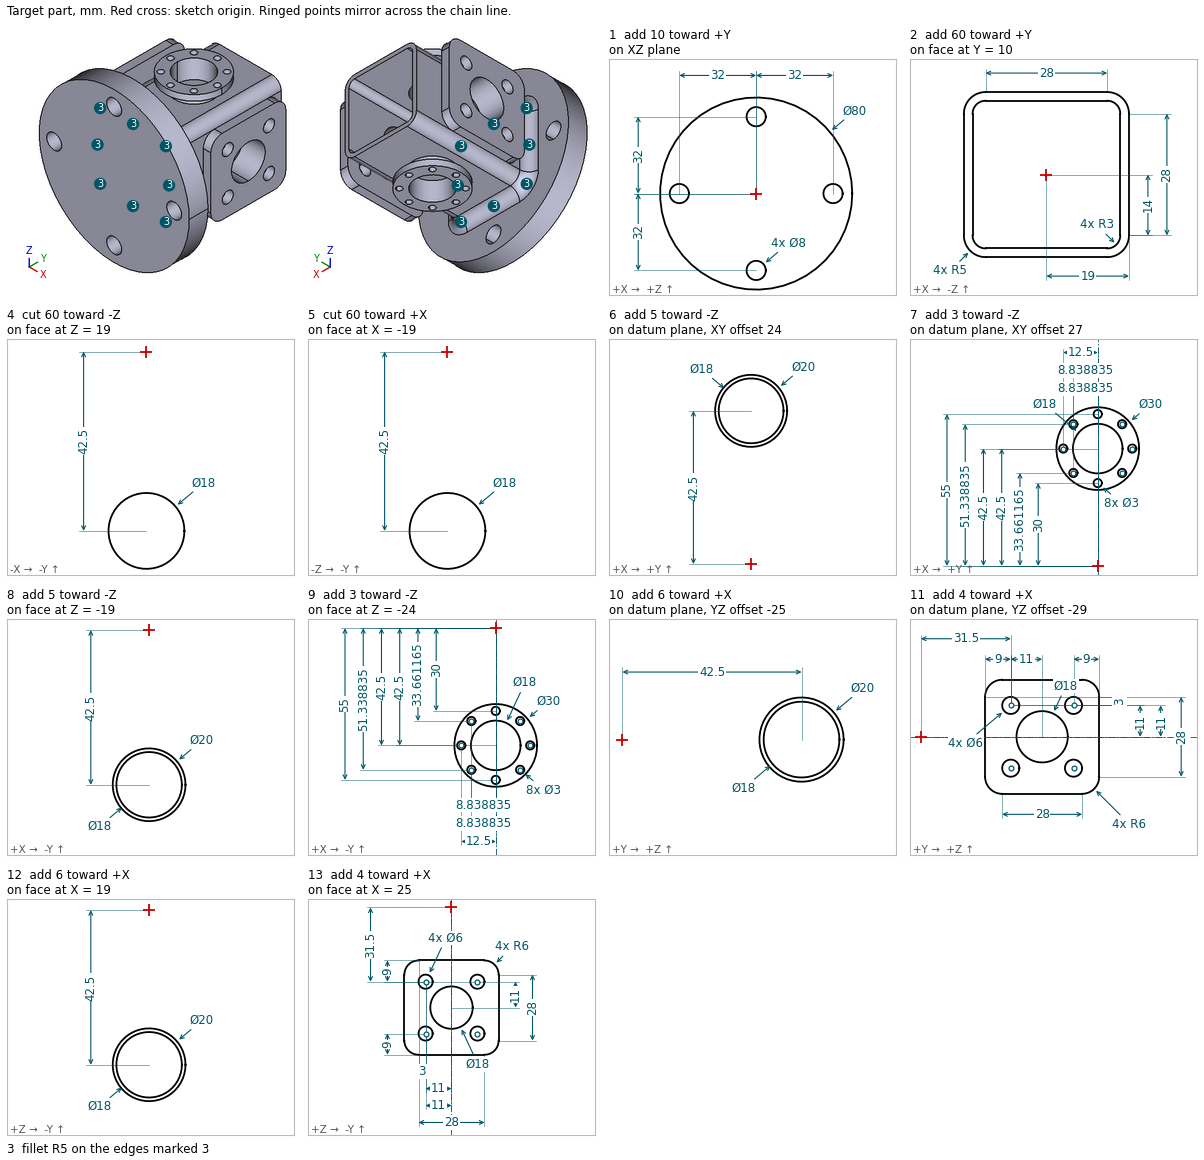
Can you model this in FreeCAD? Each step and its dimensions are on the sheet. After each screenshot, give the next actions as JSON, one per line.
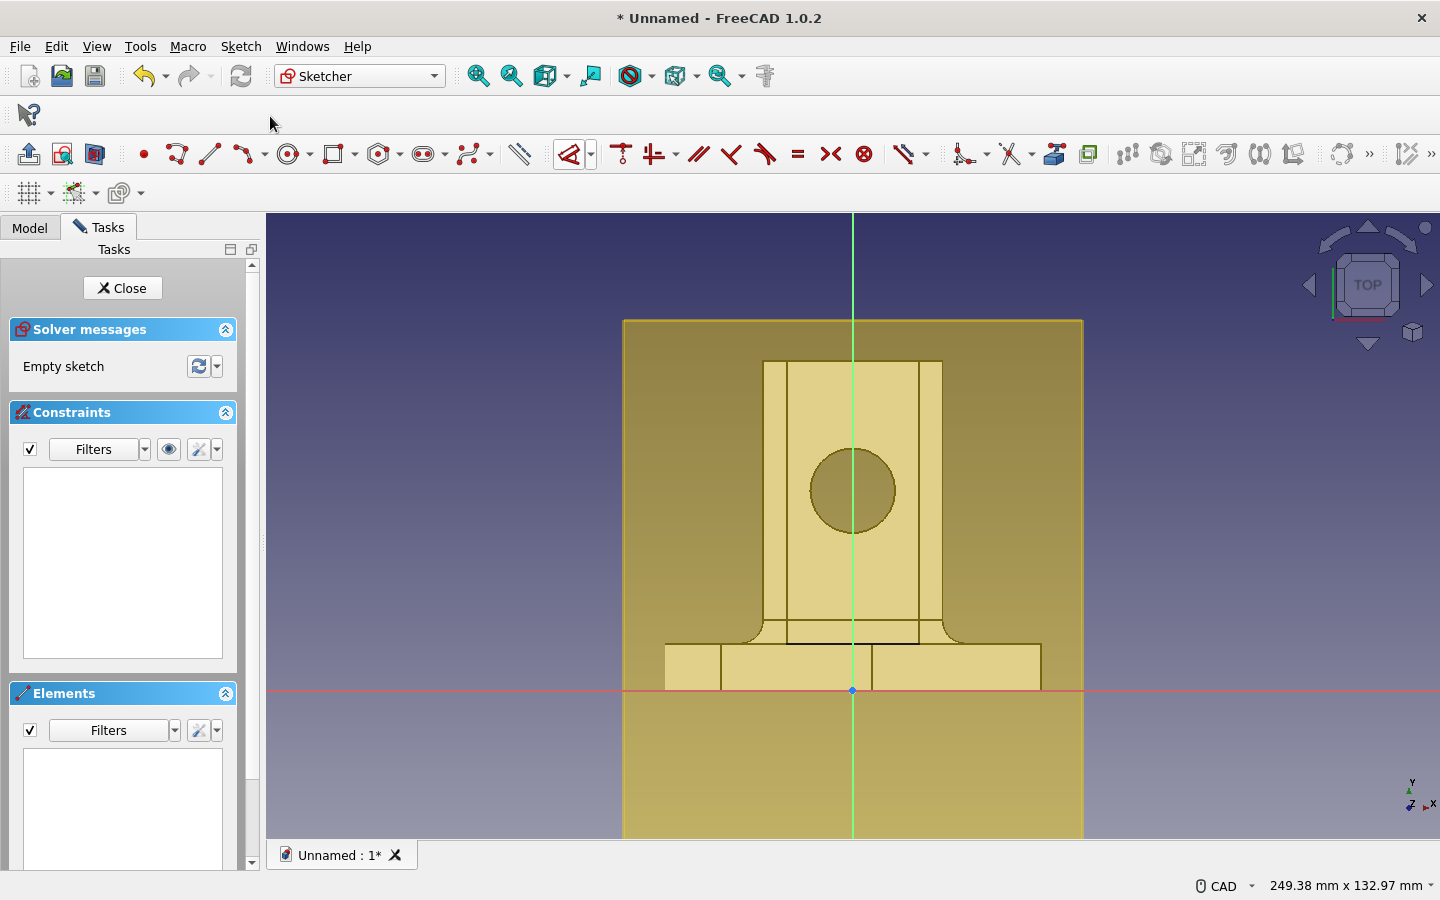
{"action": "scroll", "coordinate": [875, 479], "scroll_direction": "up", "scroll_amount": 7}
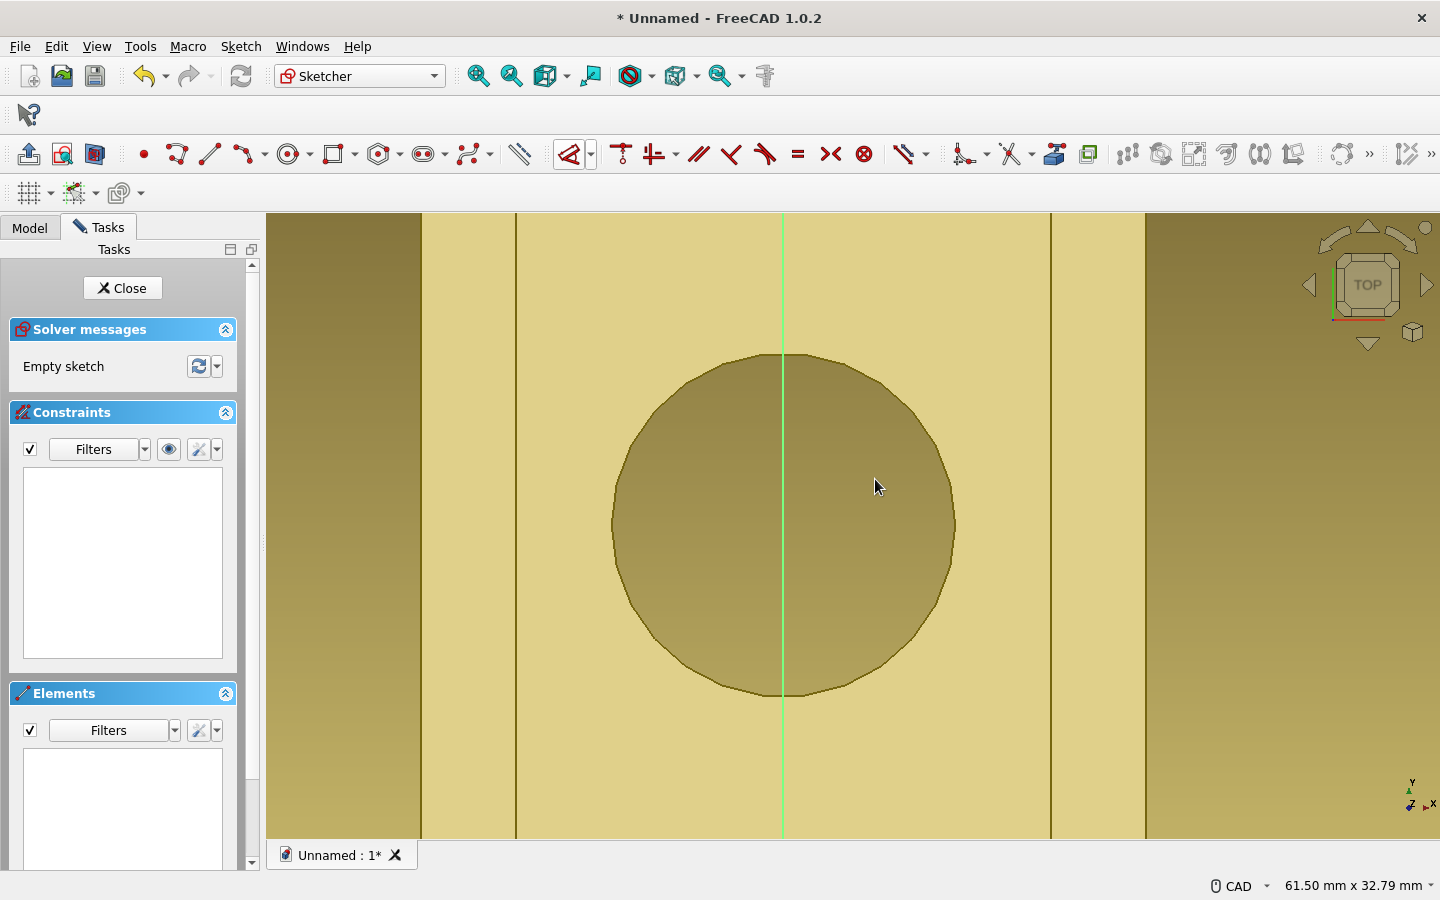
{"action": "key", "text": "g c"}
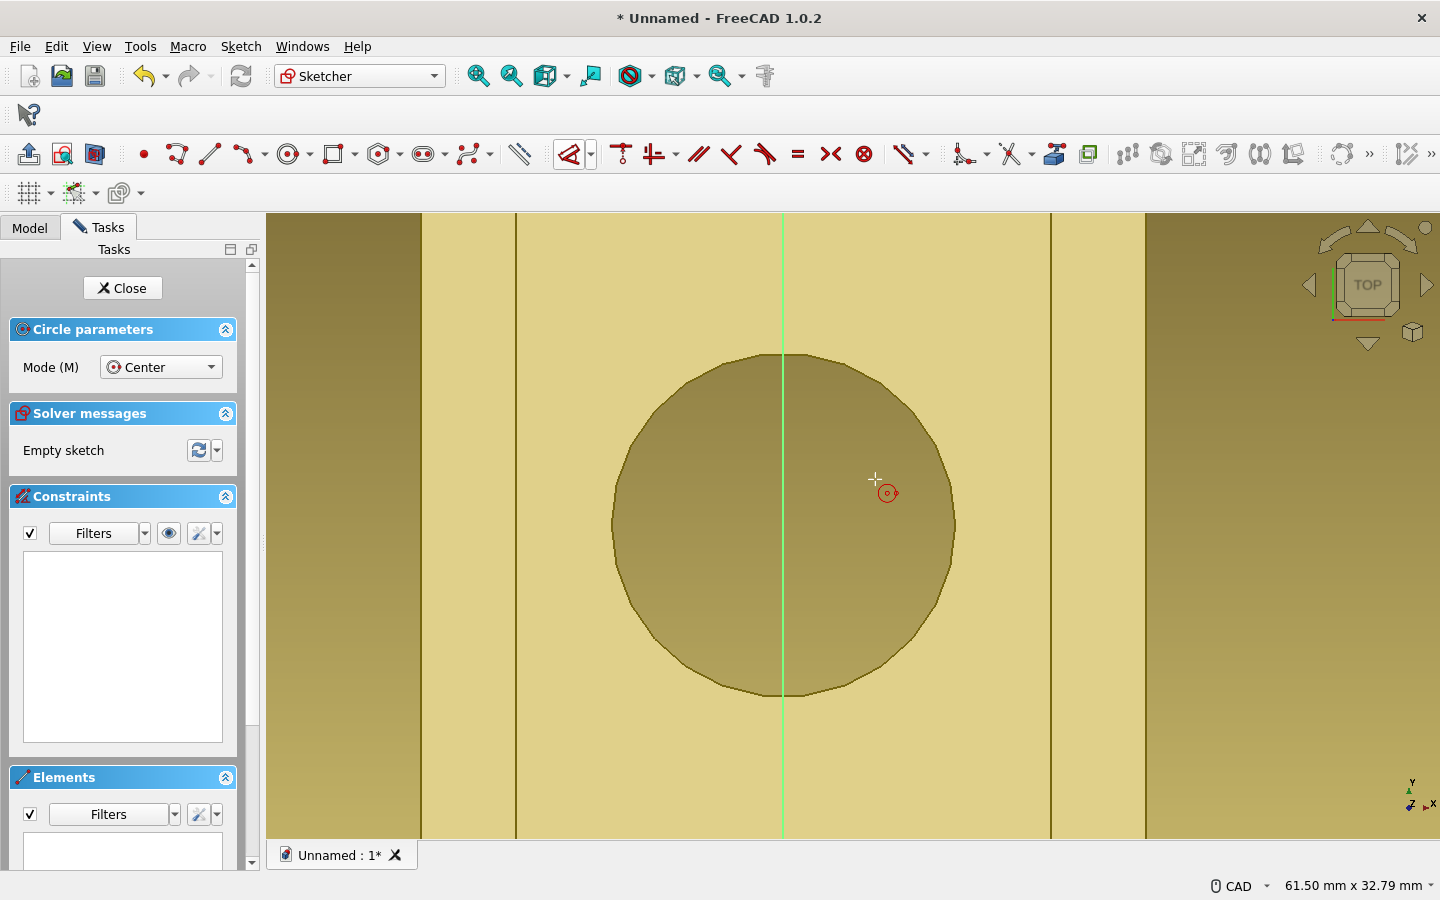
{"action": "left_click", "coordinate": [783, 525]}
{"action": "mouse_move", "coordinate": [918, 390]}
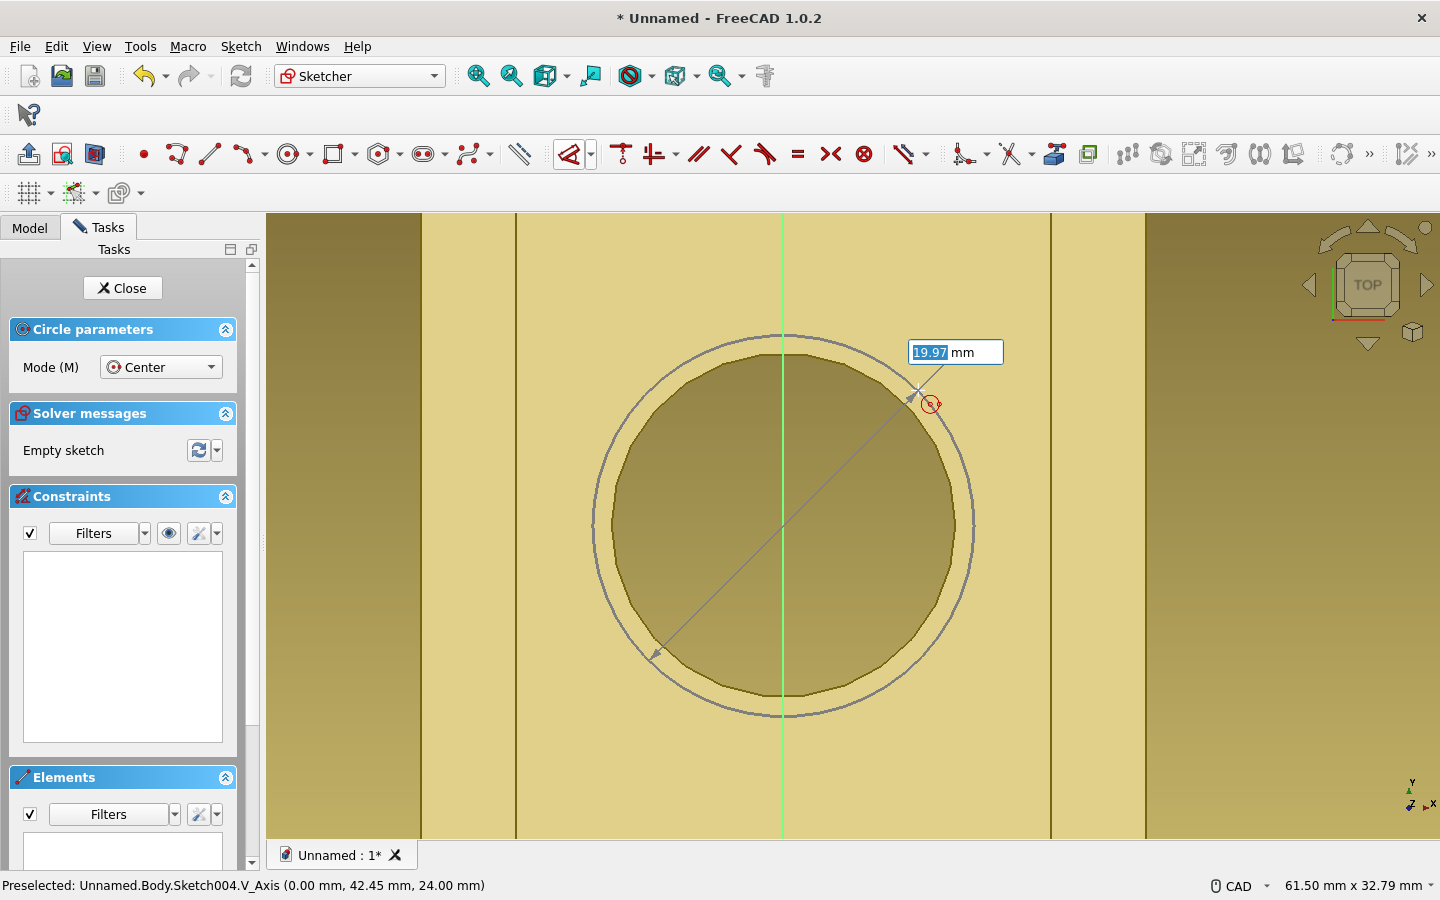
{"action": "type", "text": "20"}
{"action": "key", "text": "Return"}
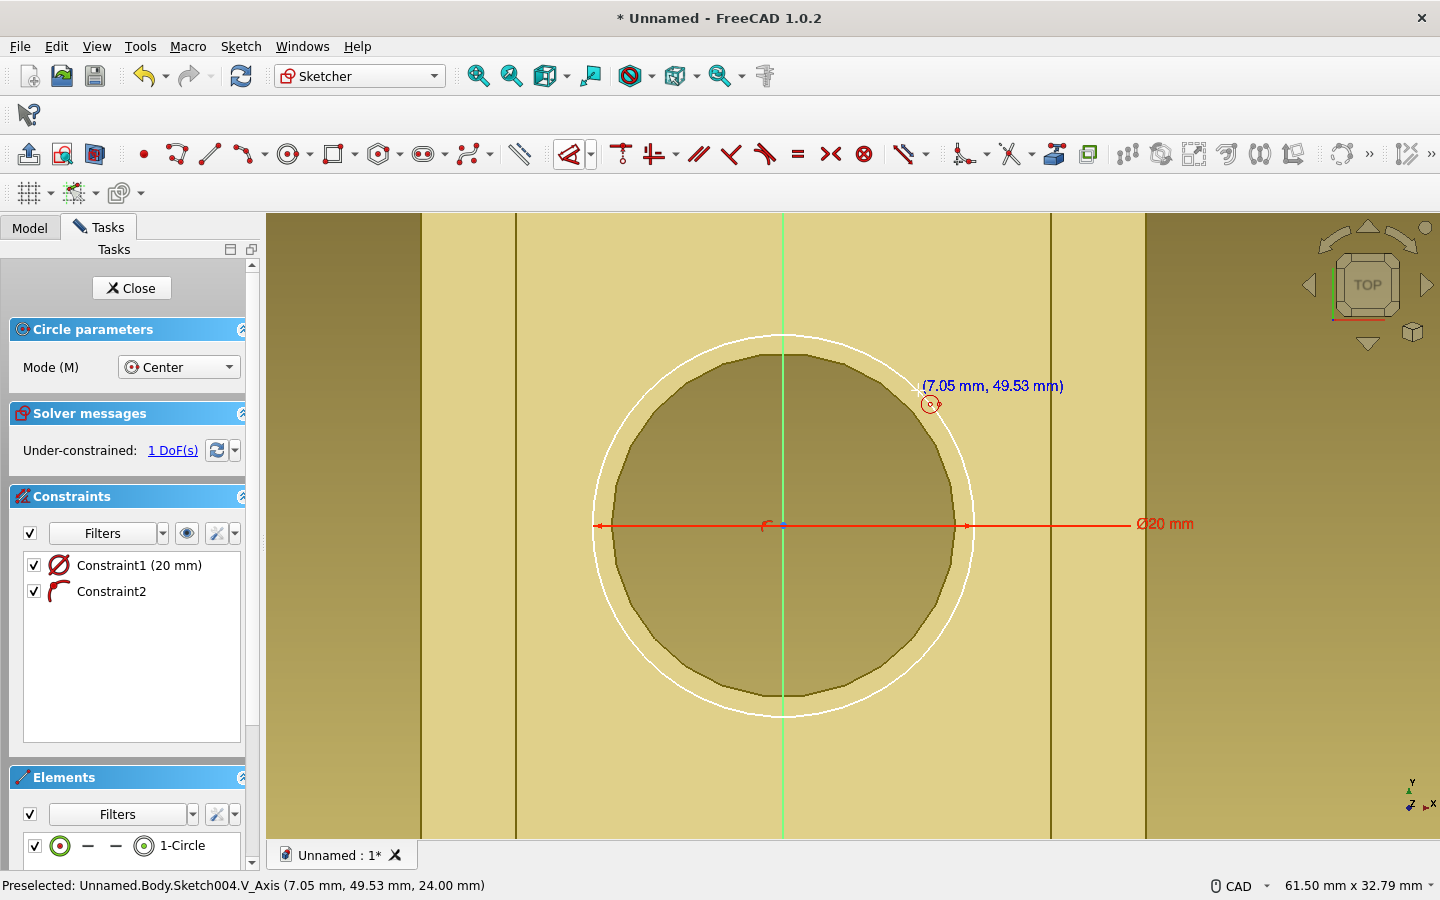
{"action": "left_click", "coordinate": [783, 526]}
{"action": "mouse_move", "coordinate": [905, 404]}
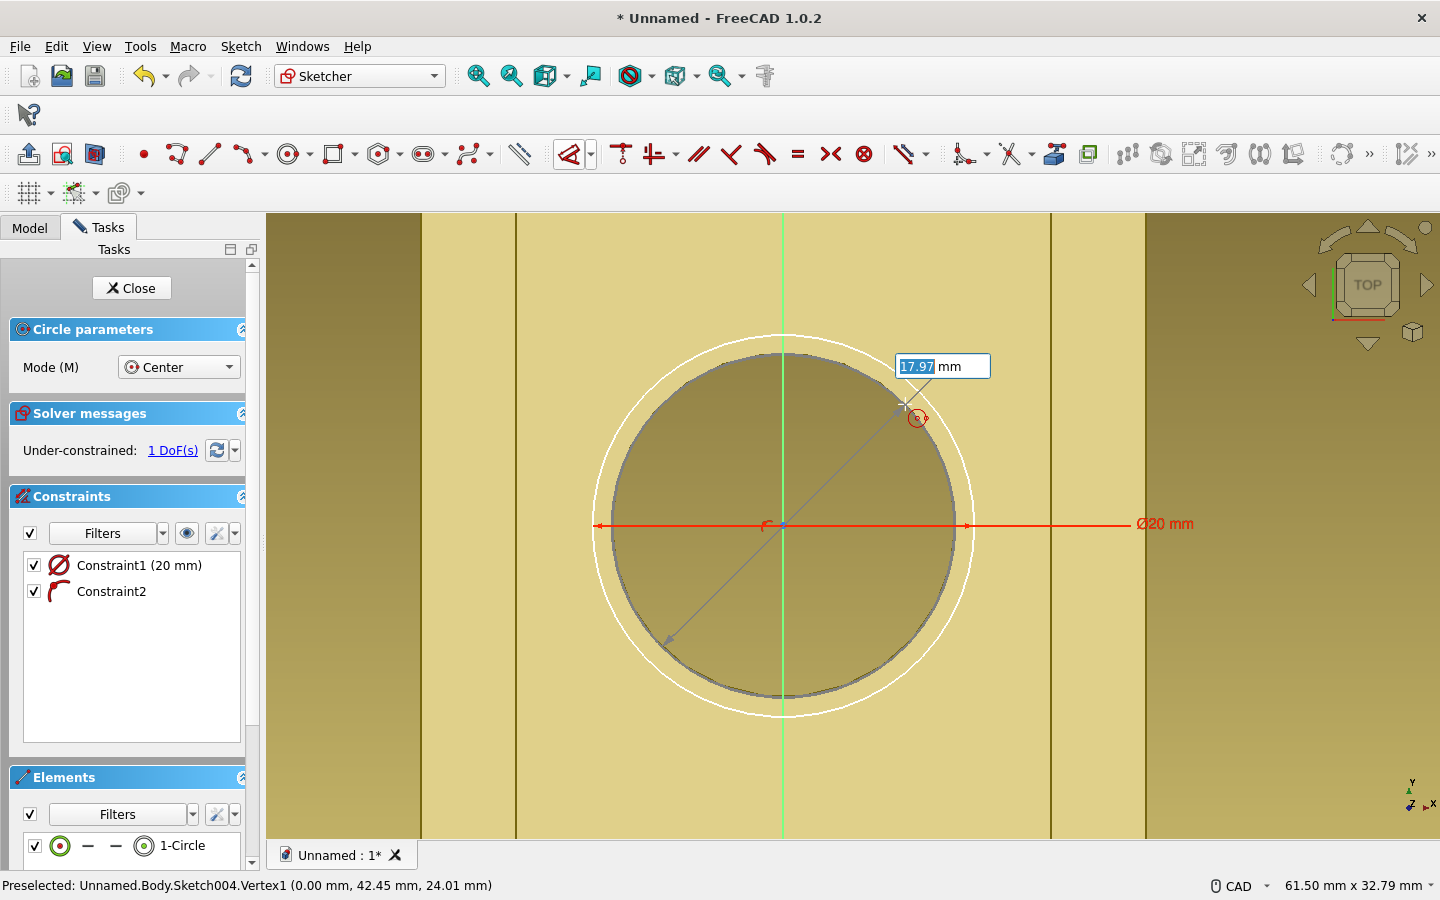
{"action": "type", "text": "18"}
{"action": "key", "text": "Return"}
{"action": "key", "text": "Escape"}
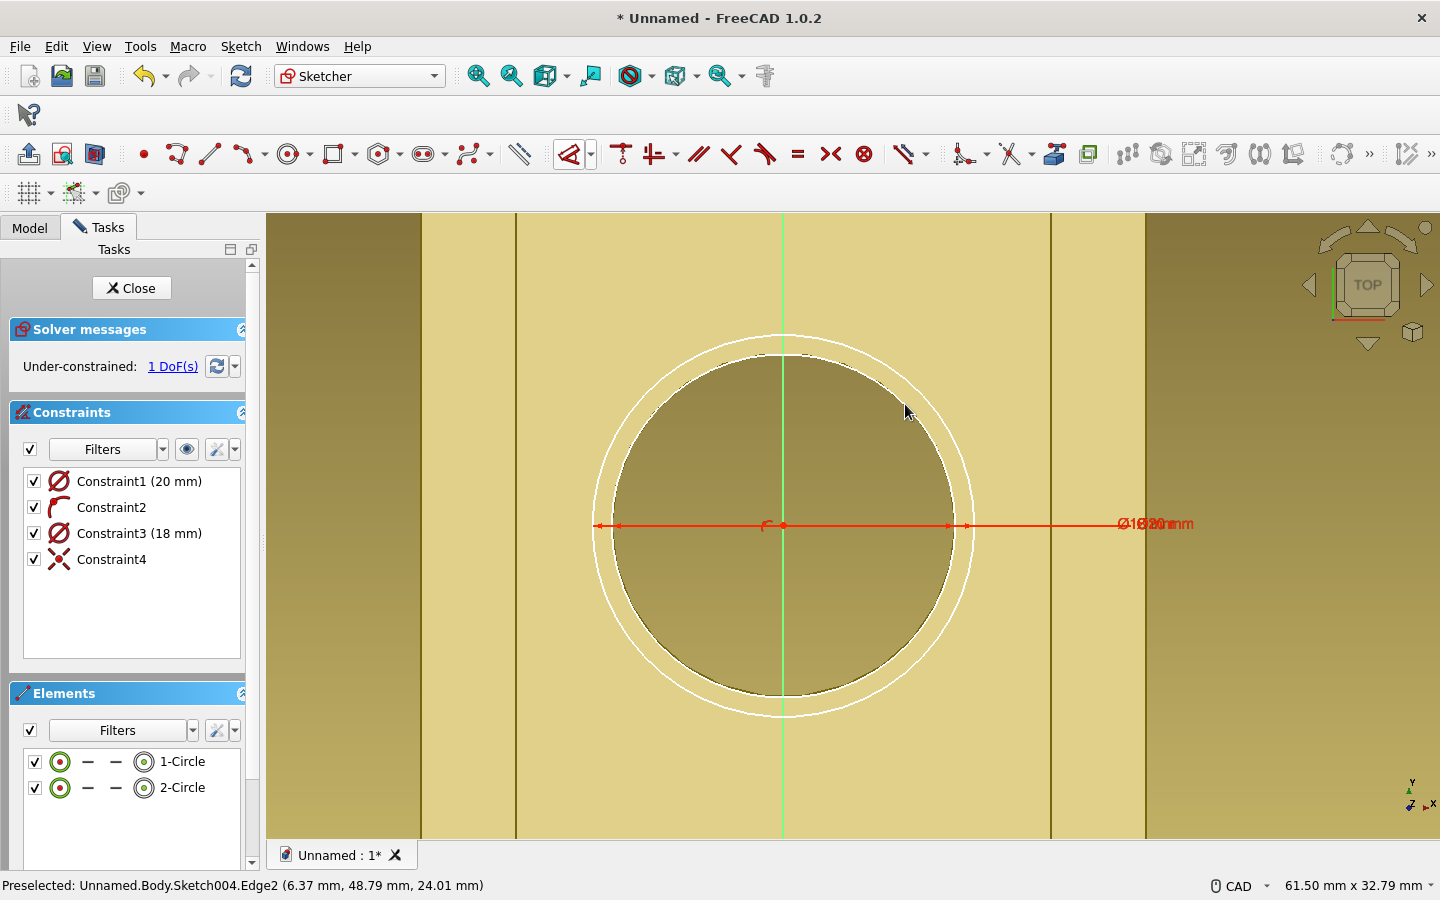
{"action": "left_click", "coordinate": [783, 526]}